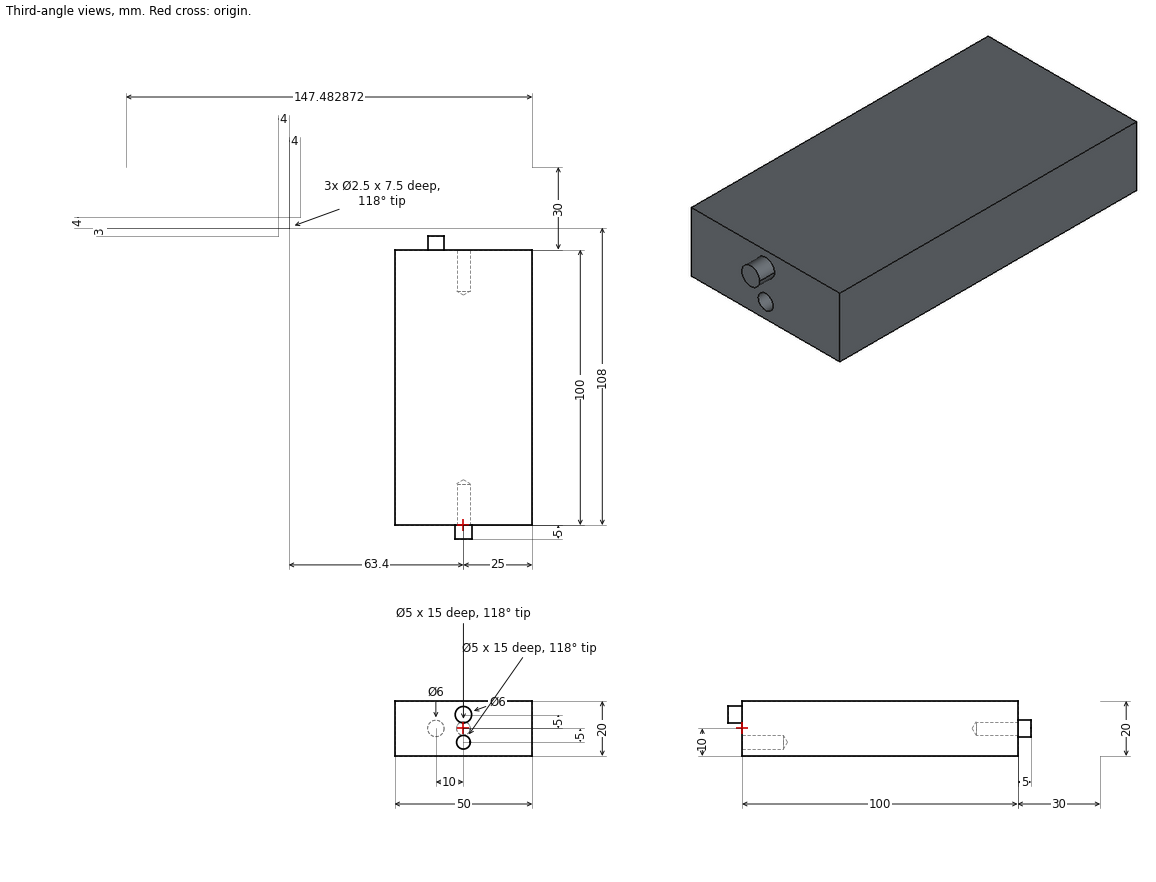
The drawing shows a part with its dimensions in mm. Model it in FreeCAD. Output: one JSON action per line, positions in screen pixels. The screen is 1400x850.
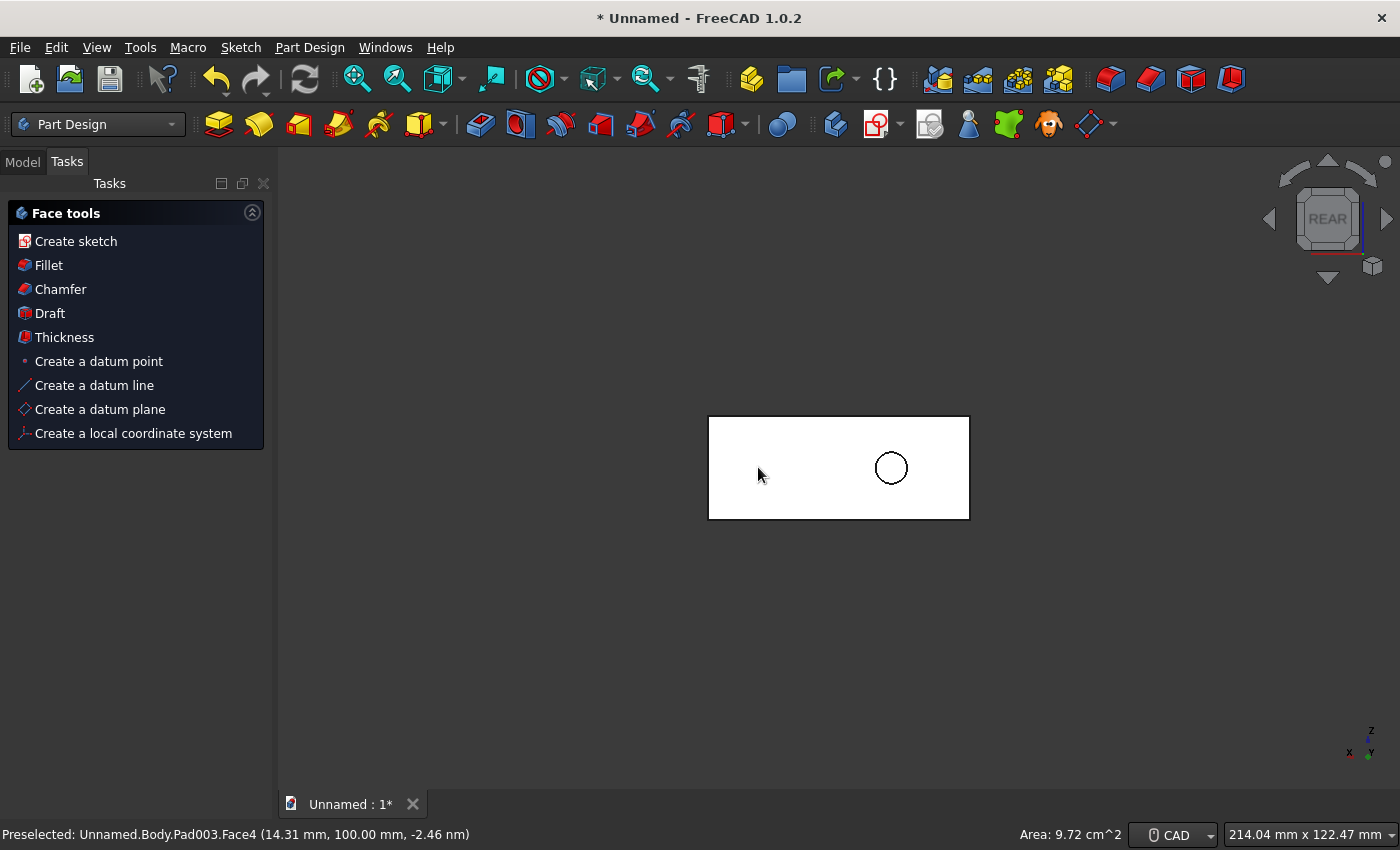
{"action": "left_click", "coordinate": [876, 124]}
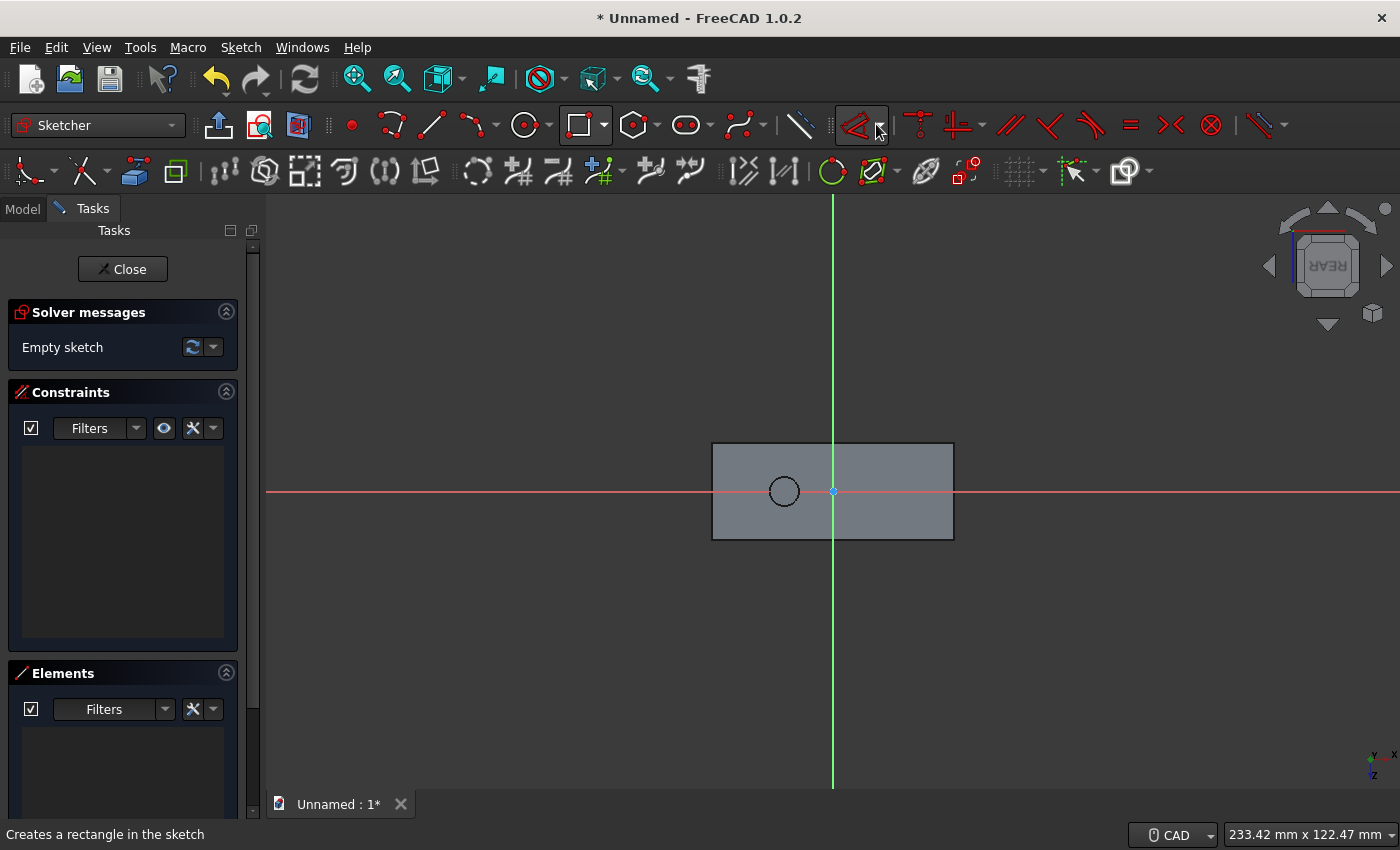
{"action": "scroll", "coordinate": [837, 491], "scroll_direction": "up", "scroll_amount": 14}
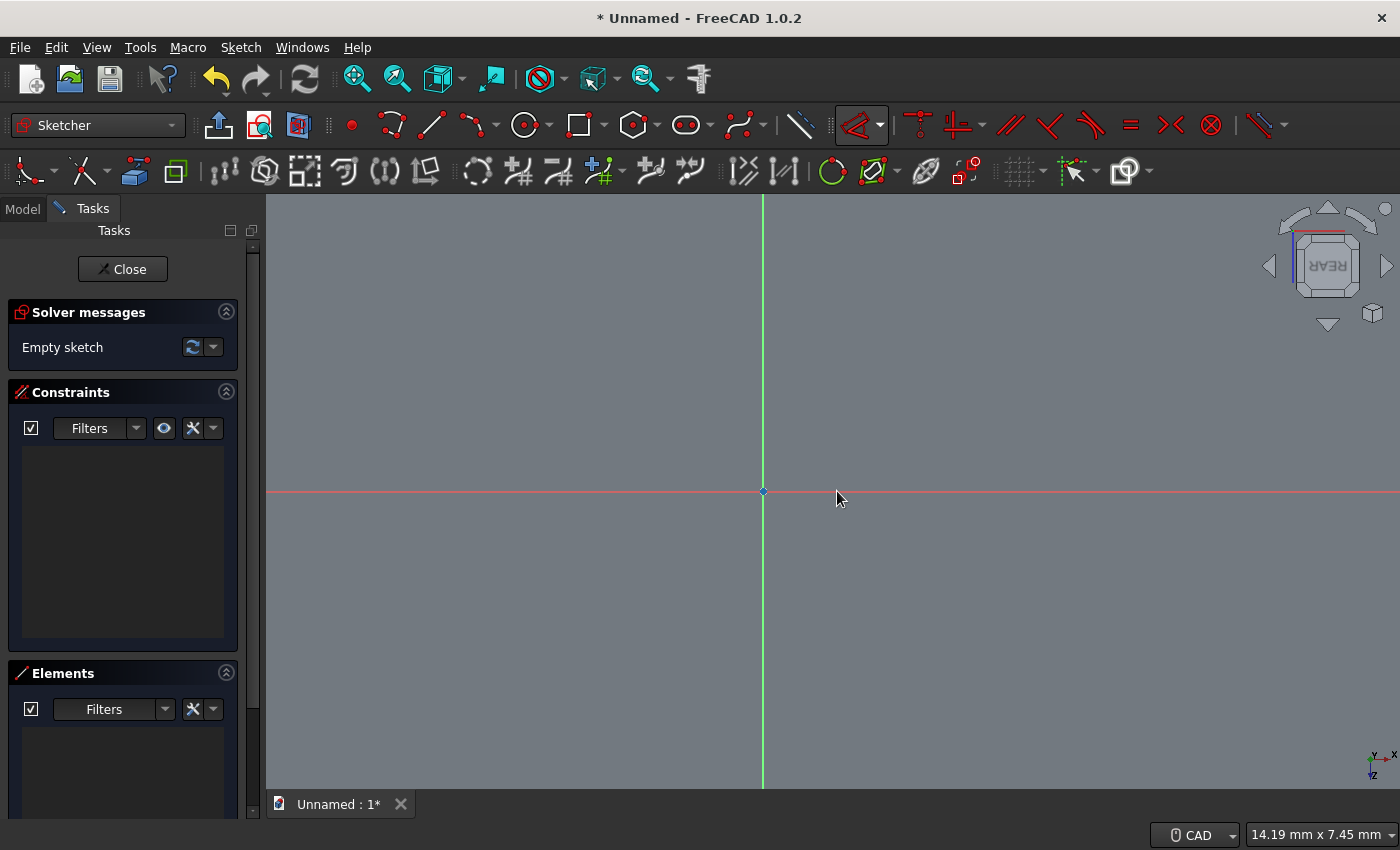
{"action": "key", "text": "g c"}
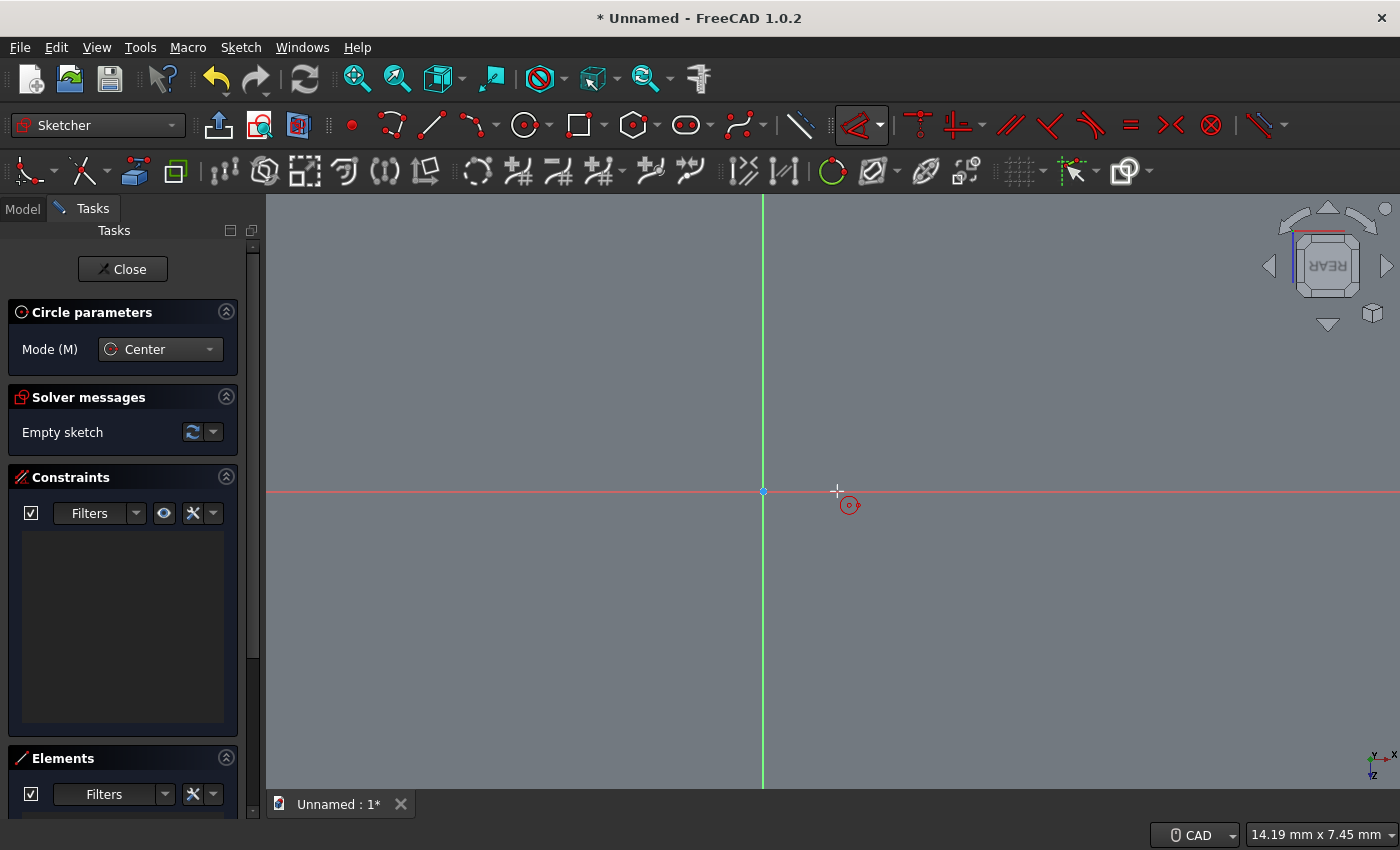
{"action": "left_click", "coordinate": [763, 491]}
{"action": "left_click", "coordinate": [905, 350]}
{"action": "key", "text": "Escape"}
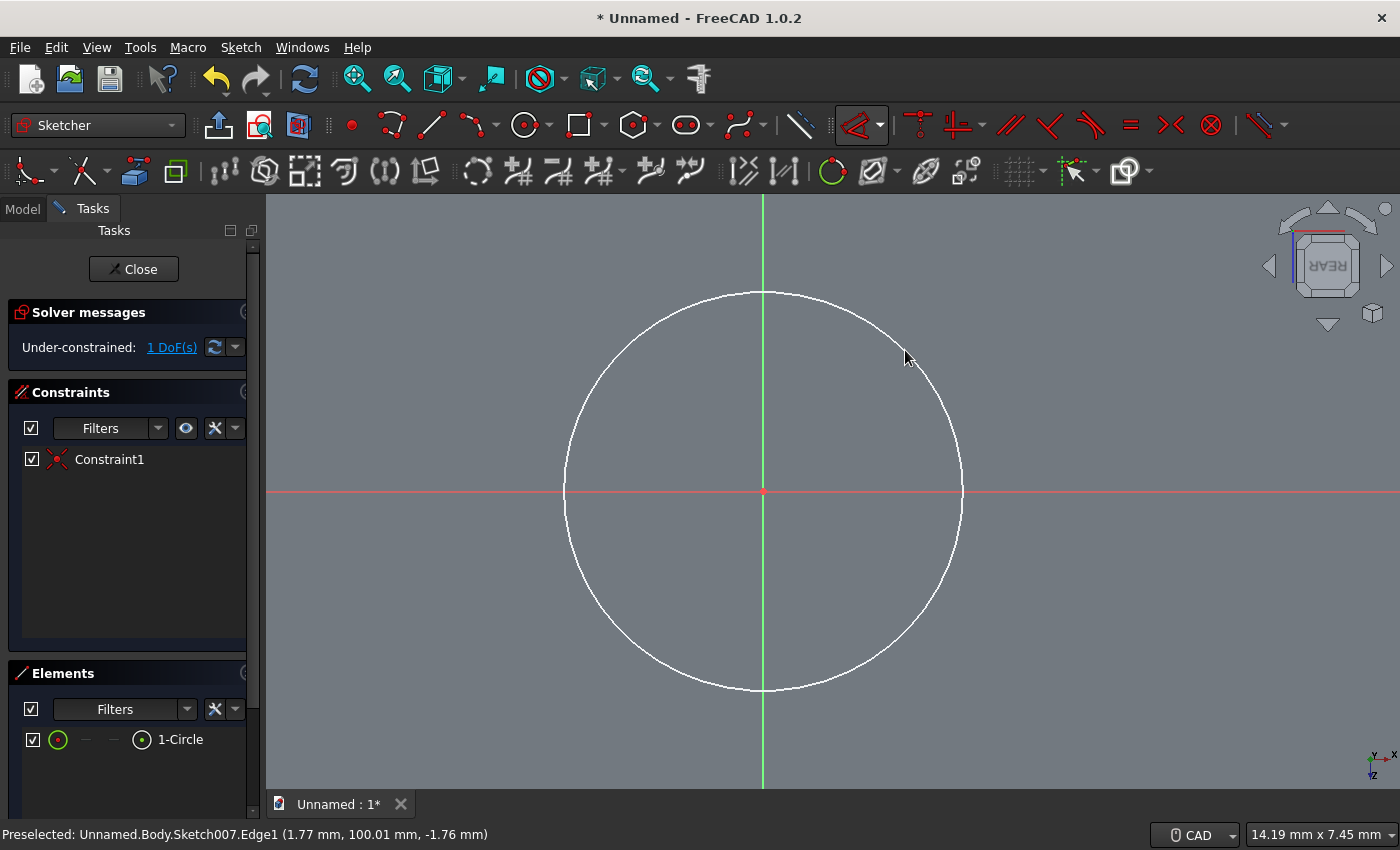
{"action": "left_click", "coordinate": [904, 350]}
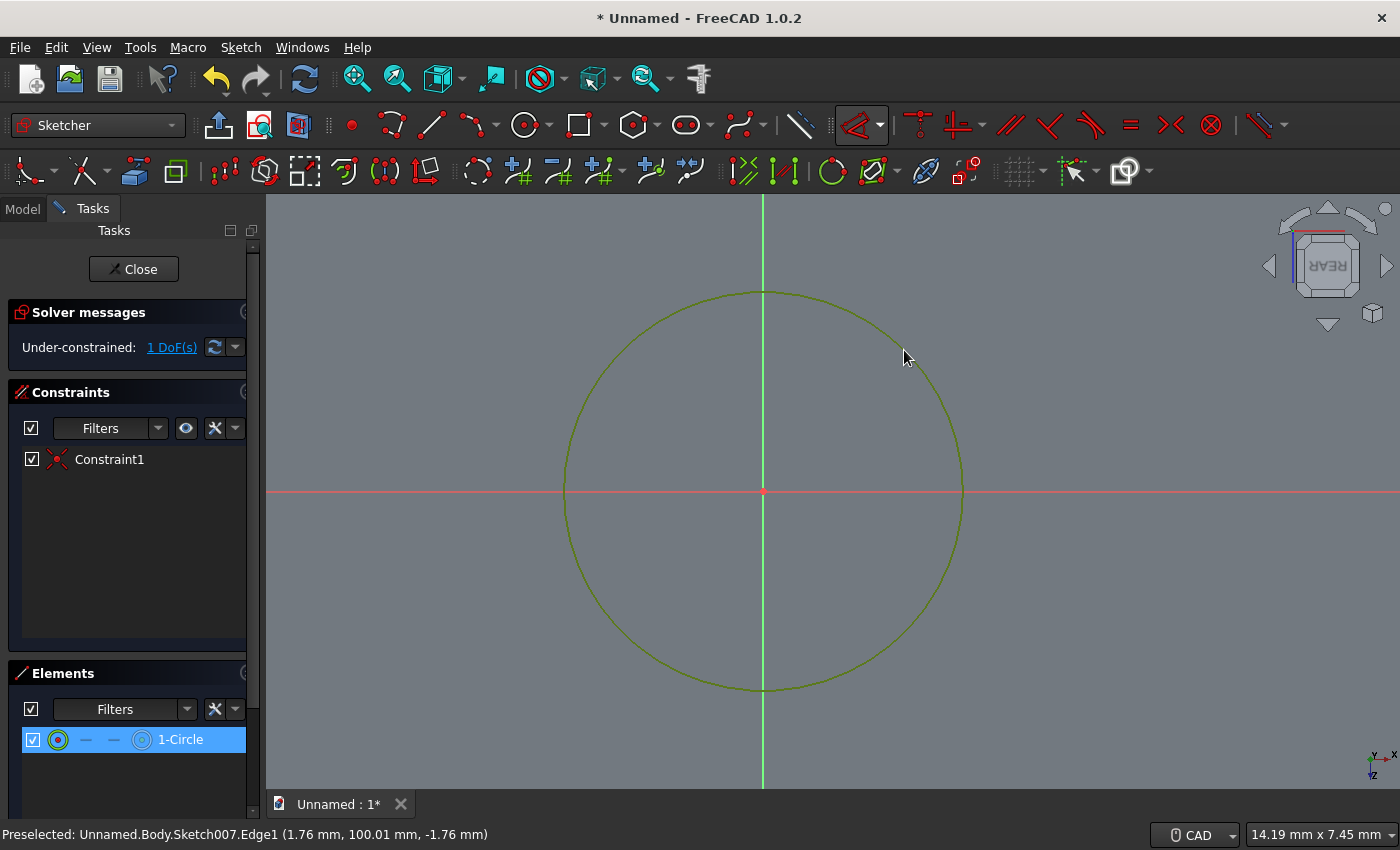
{"action": "key", "text": "k o"}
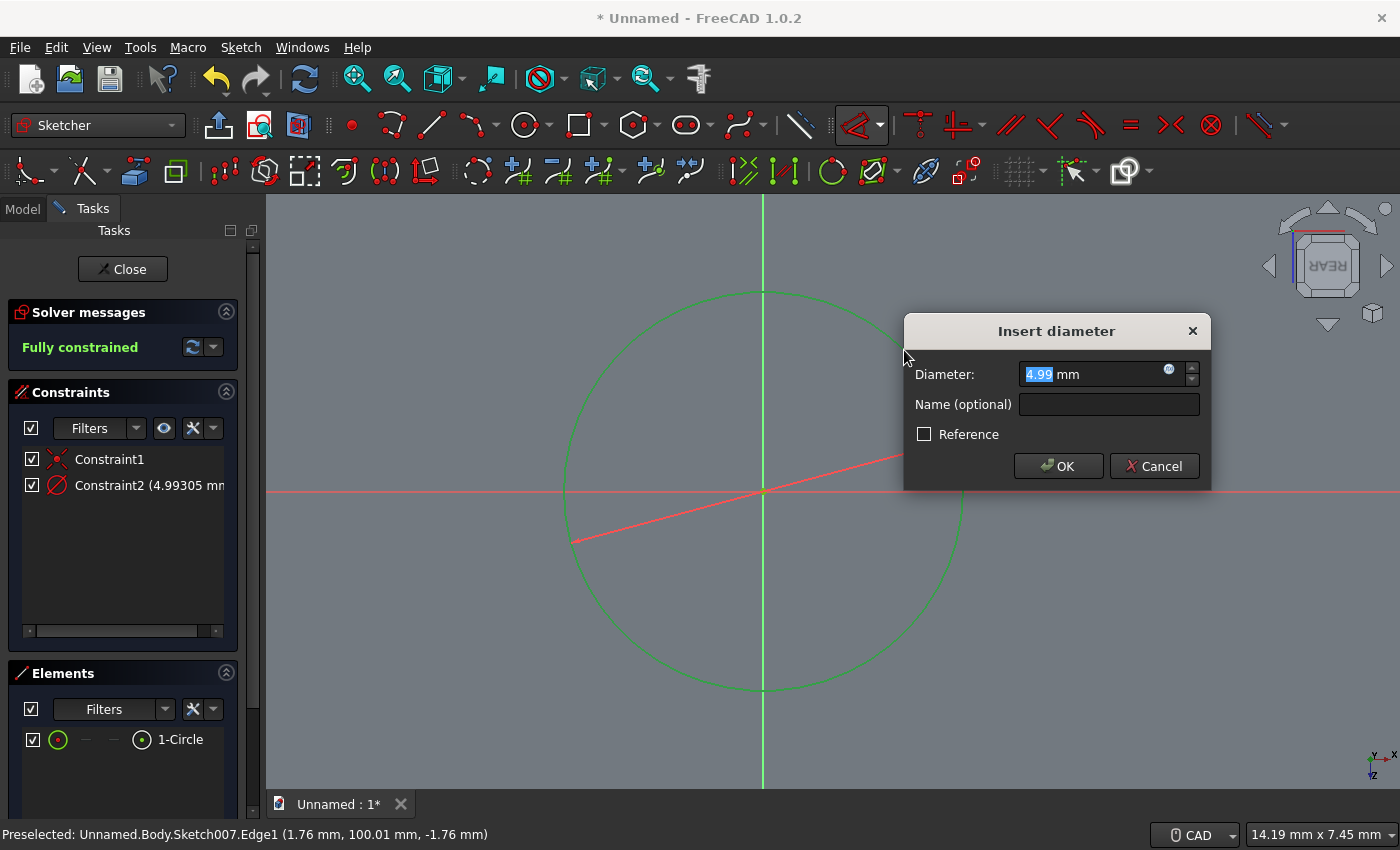
{"action": "type", "text": "5"}
{"action": "key", "text": "Return"}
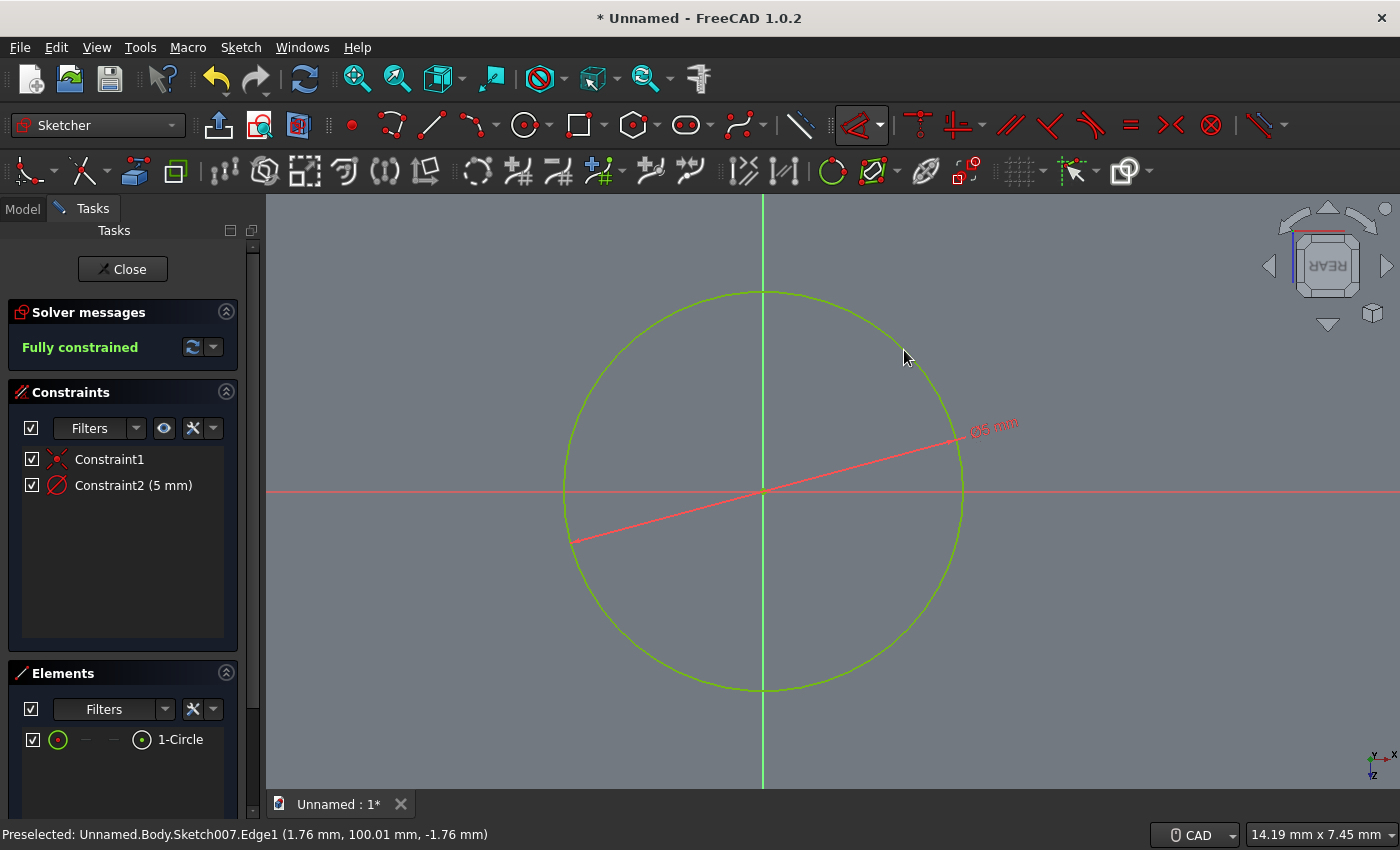
{"action": "left_click", "coordinate": [123, 269]}